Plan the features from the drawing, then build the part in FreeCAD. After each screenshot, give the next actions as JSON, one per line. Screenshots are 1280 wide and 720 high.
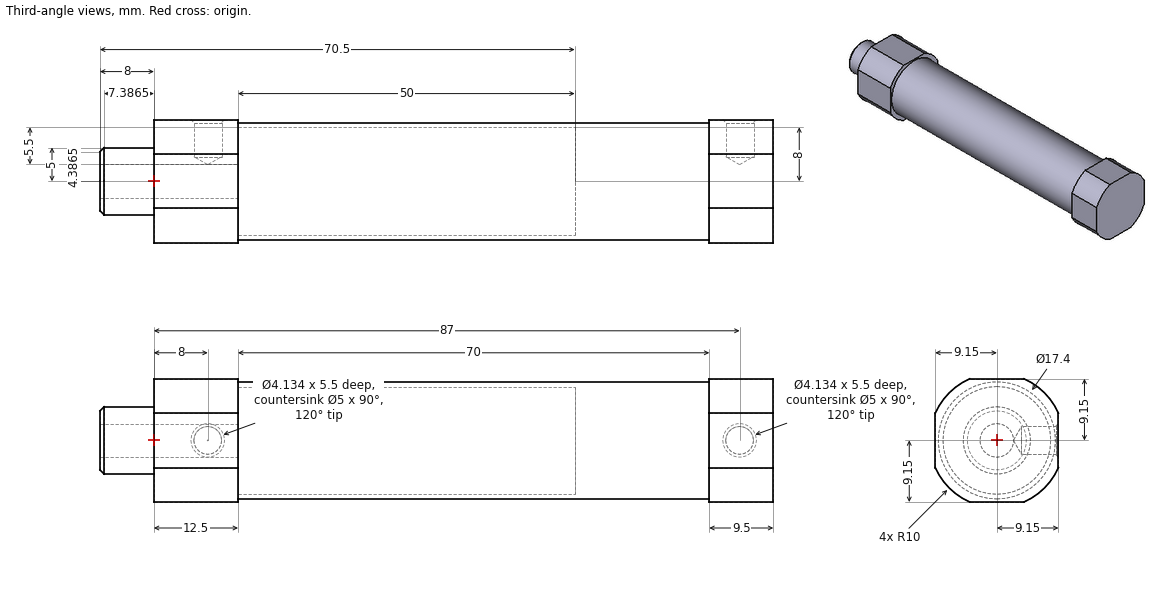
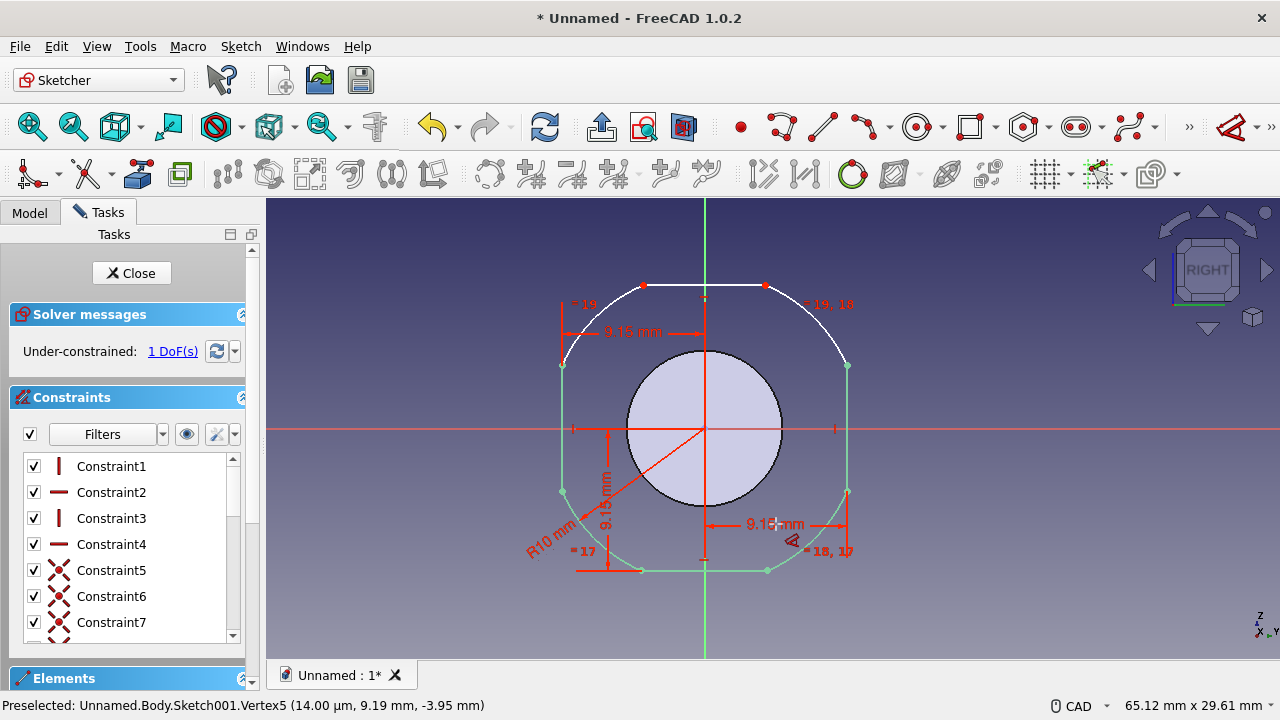
{"action": "left_click", "coordinate": [766, 285]}
{"action": "left_click", "coordinate": [800, 357]}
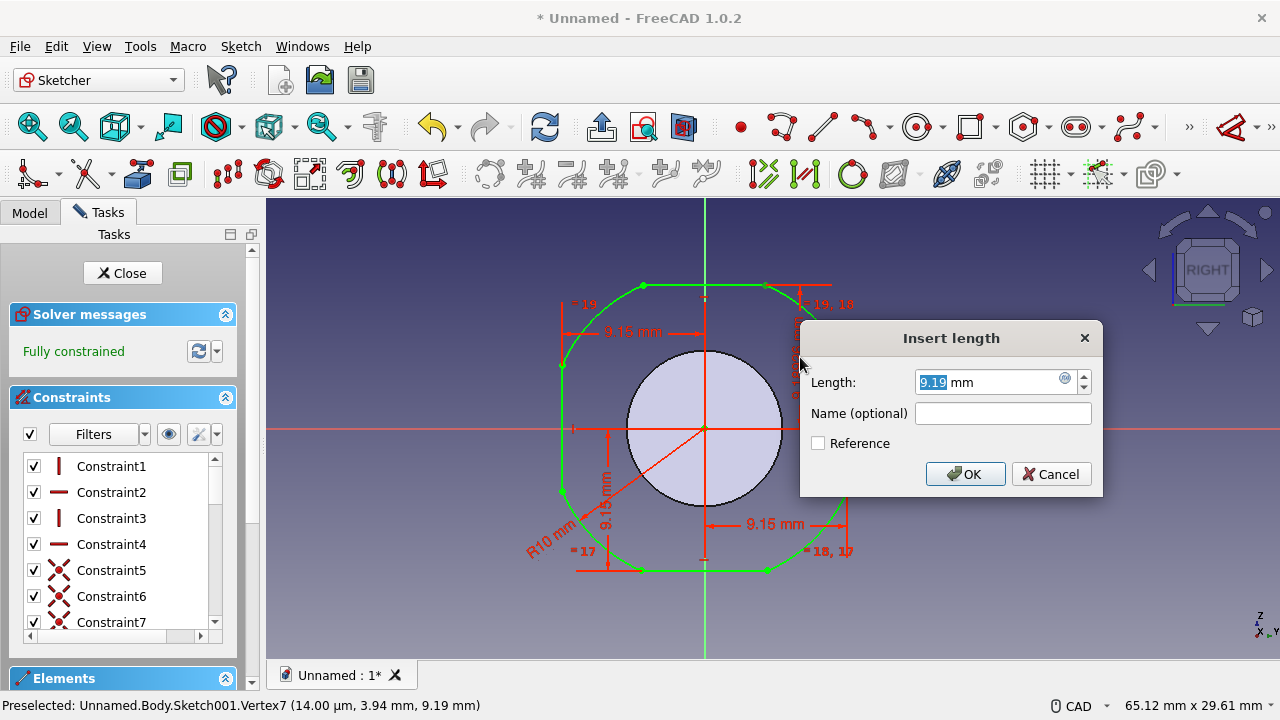
{"action": "type", "text": "9.15"}
{"action": "key", "text": "Return"}
{"action": "key", "text": "Escape"}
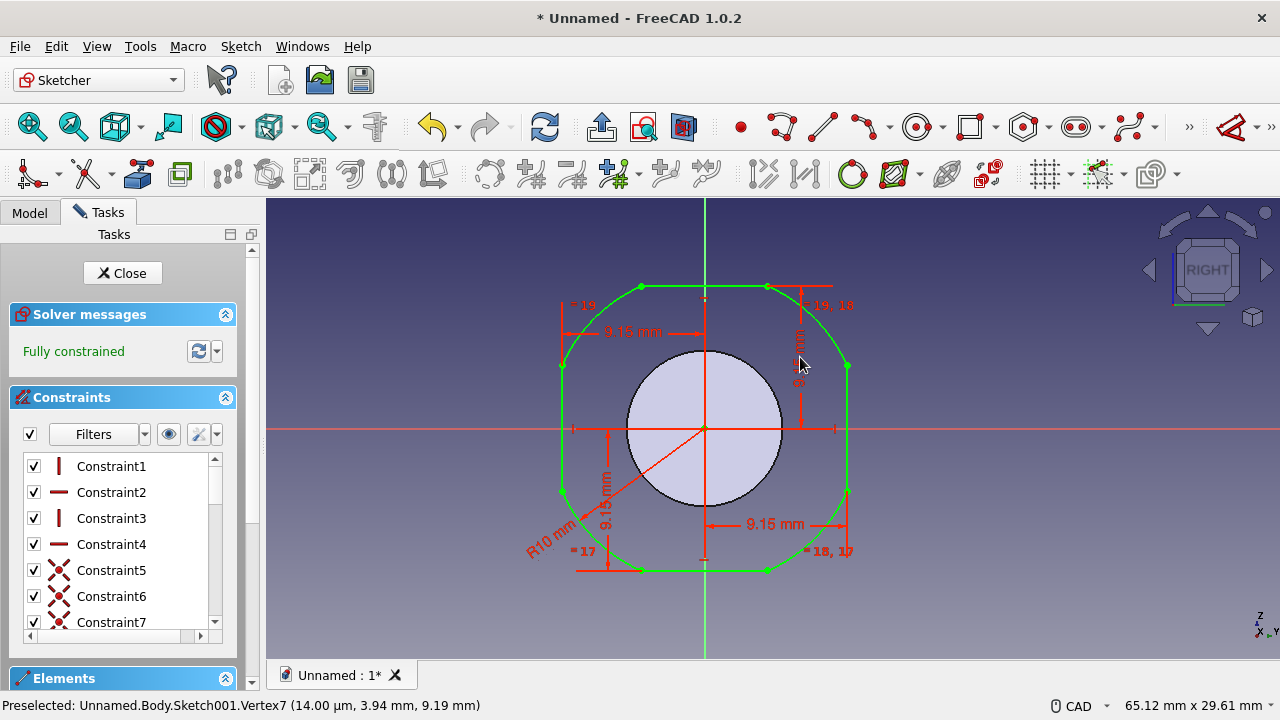
{"action": "left_click", "coordinate": [123, 273]}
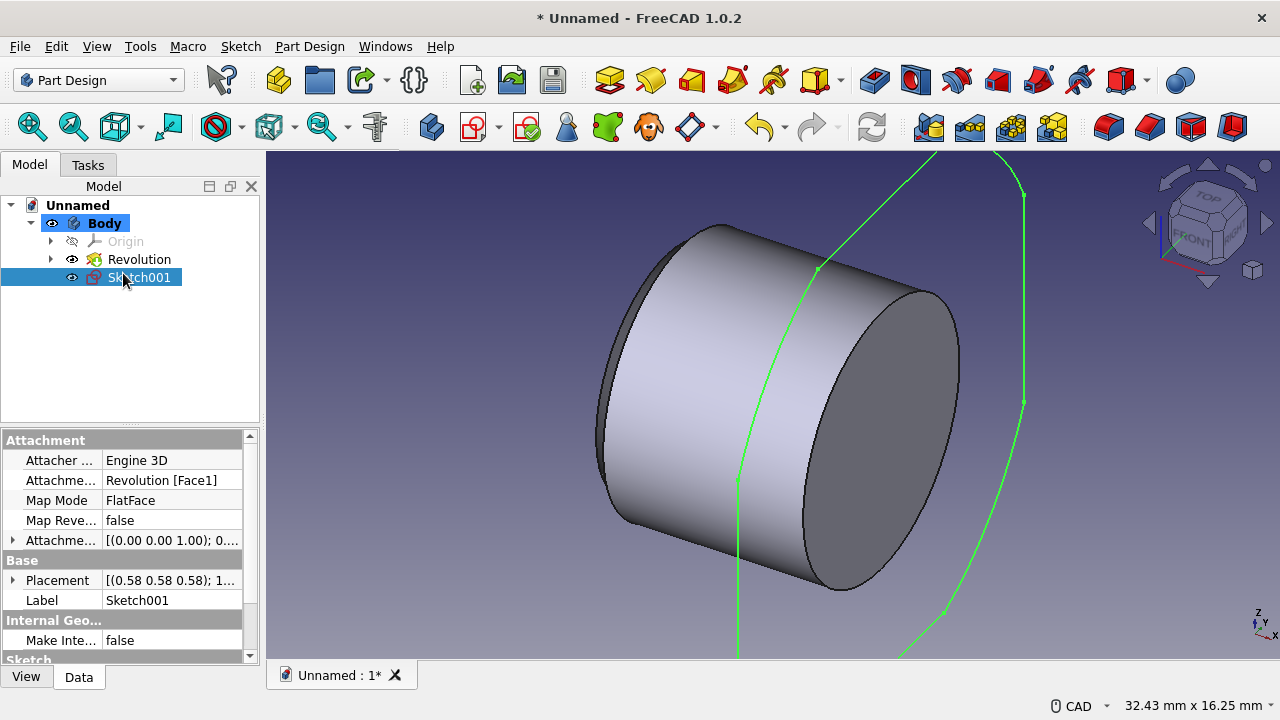
{"action": "left_click", "coordinate": [610, 80]}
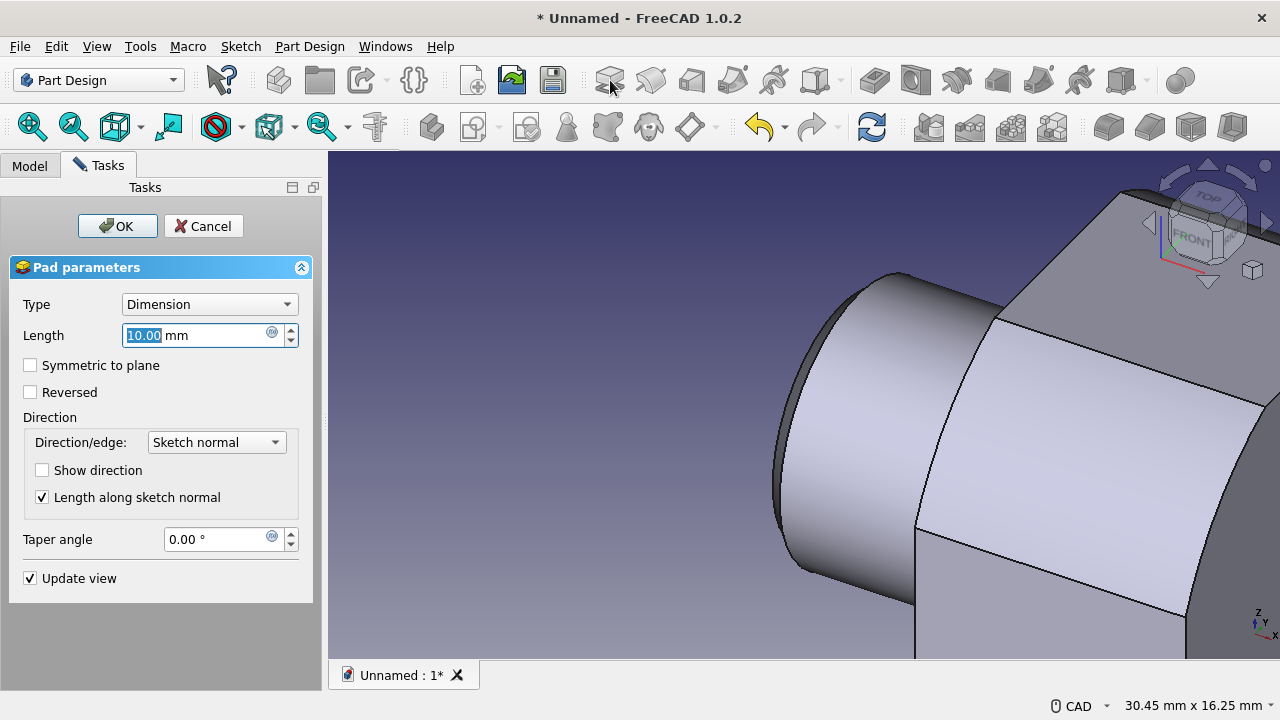
{"action": "type", "text": "12.5"}
{"action": "key", "text": "Tab"}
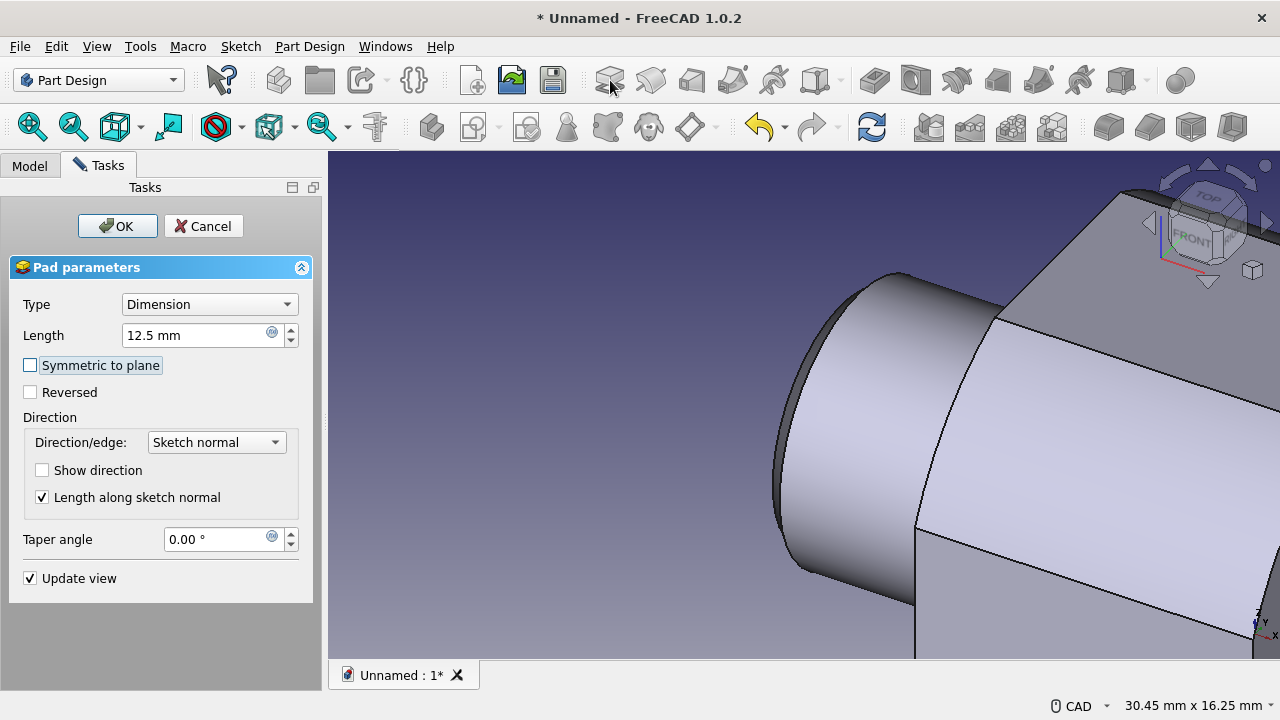
{"action": "left_click", "coordinate": [118, 226]}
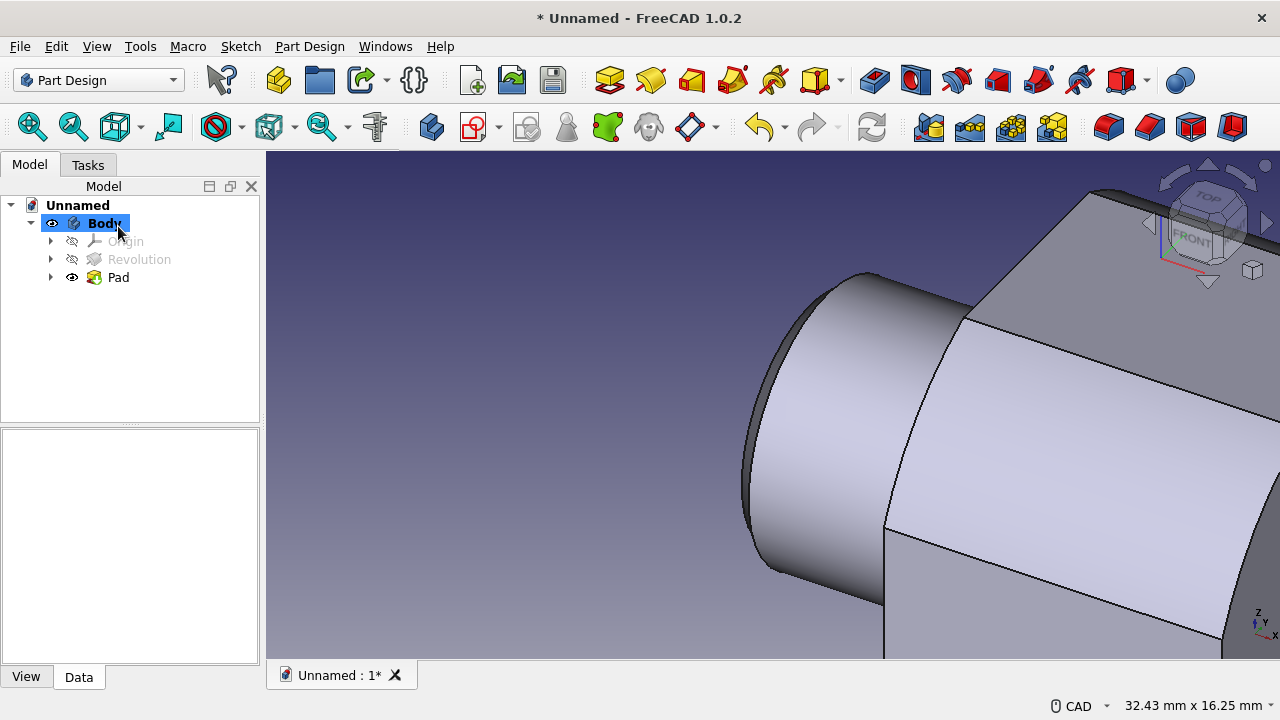
{"action": "left_click", "coordinate": [33, 128]}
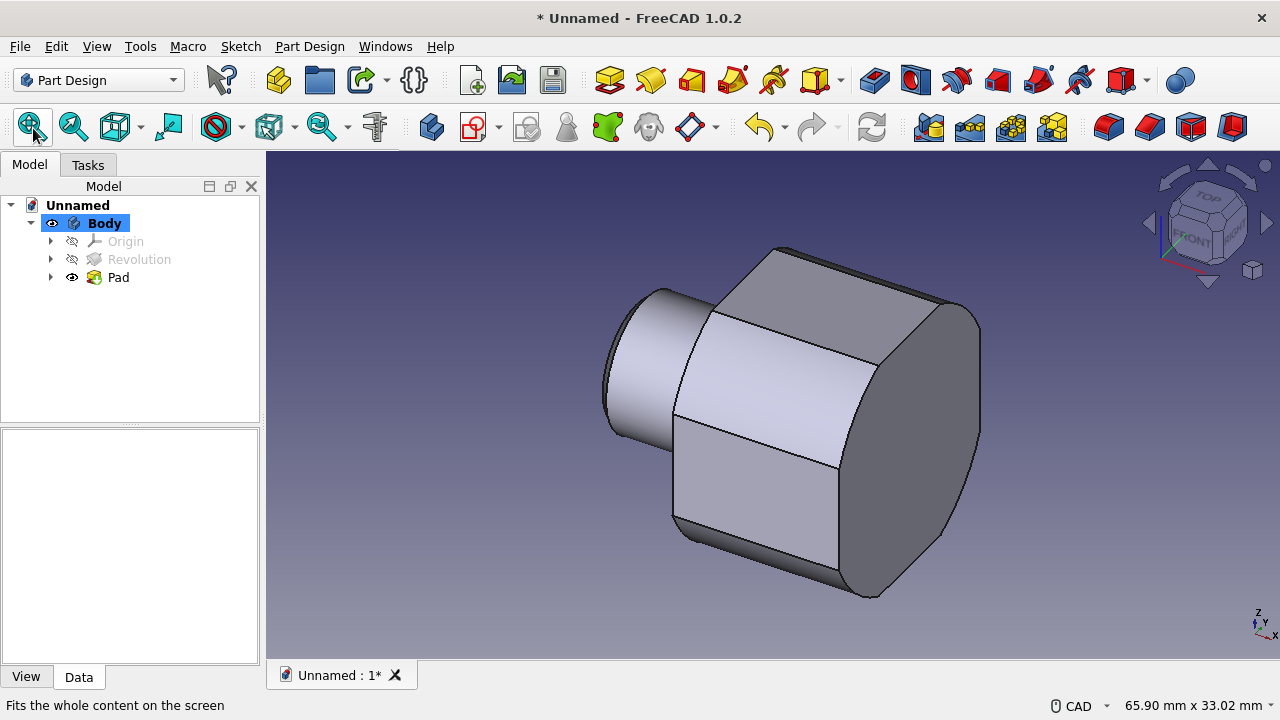
{"action": "left_click", "coordinate": [910, 449]}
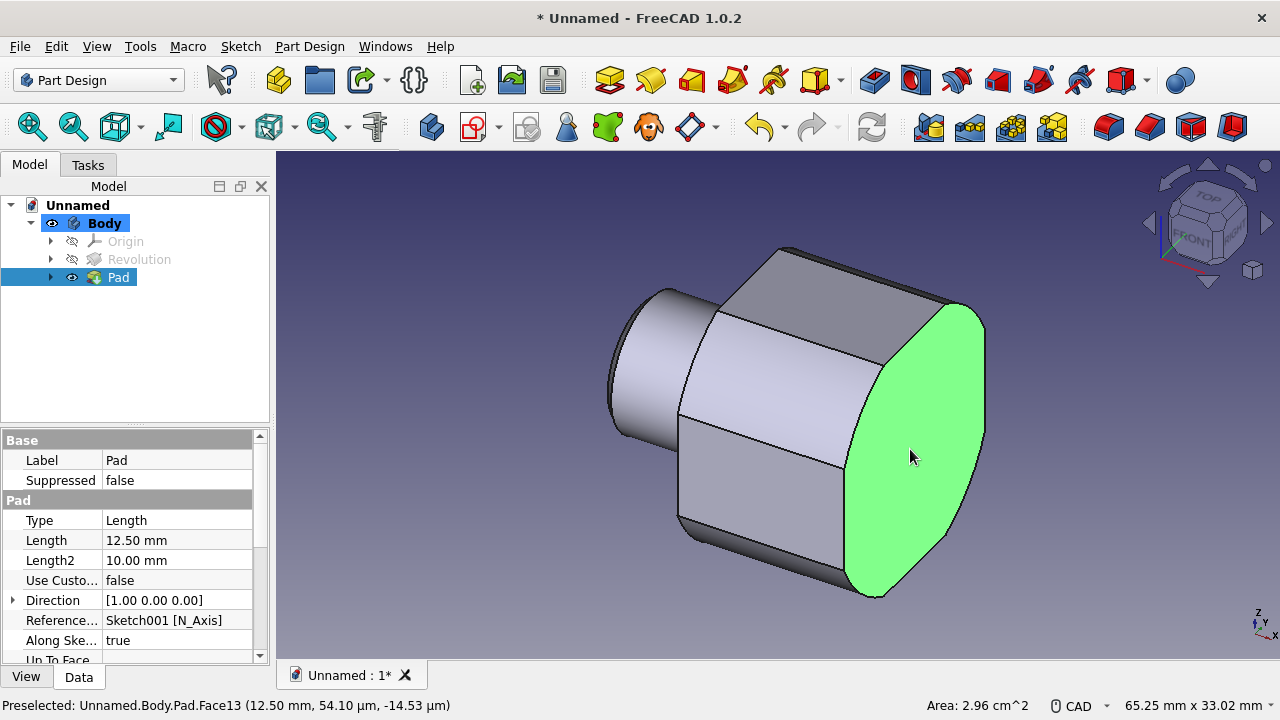
{"action": "left_click", "coordinate": [472, 128]}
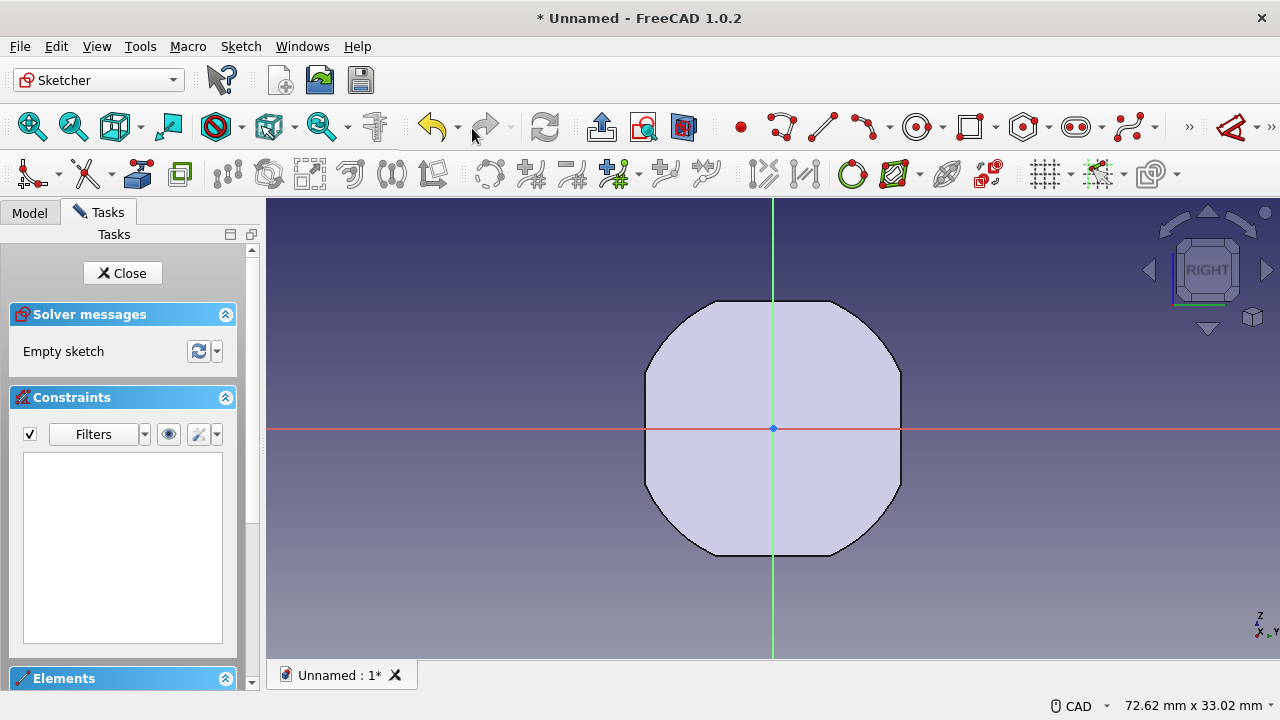
{"action": "left_click", "coordinate": [916, 128]}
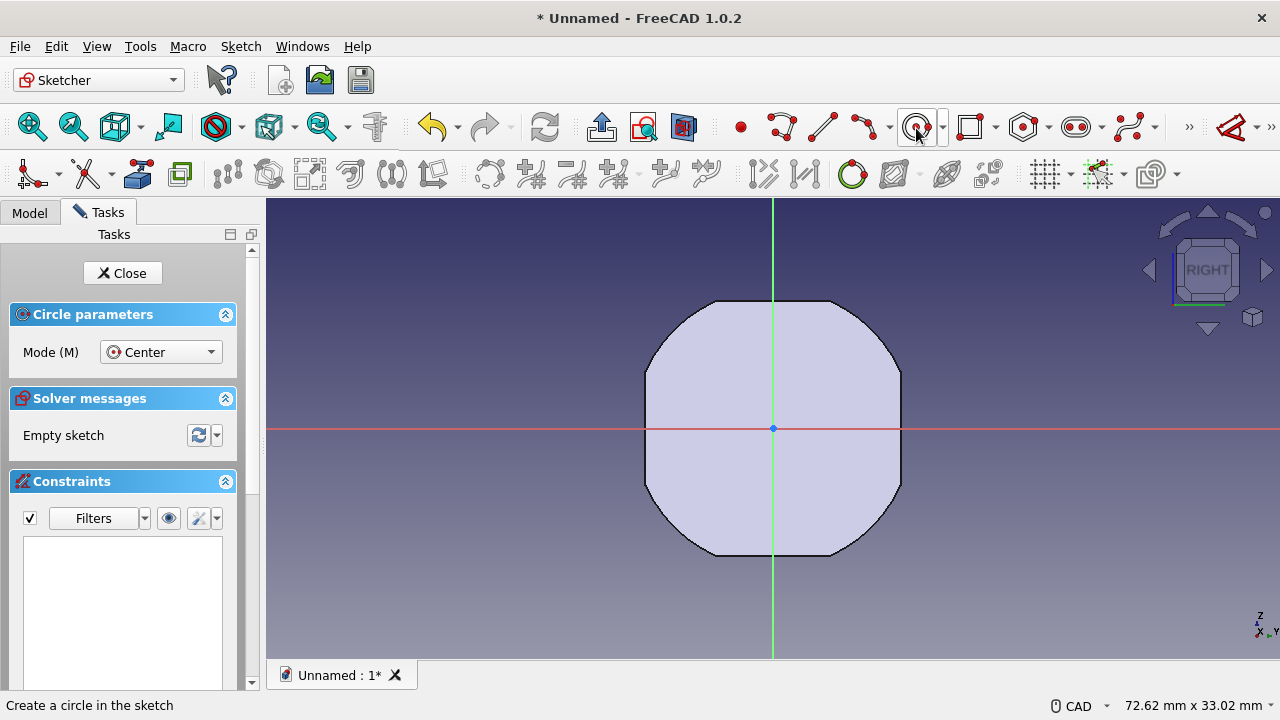
{"action": "left_click", "coordinate": [773, 428]}
{"action": "left_click", "coordinate": [859, 343]}
{"action": "key", "text": "Escape"}